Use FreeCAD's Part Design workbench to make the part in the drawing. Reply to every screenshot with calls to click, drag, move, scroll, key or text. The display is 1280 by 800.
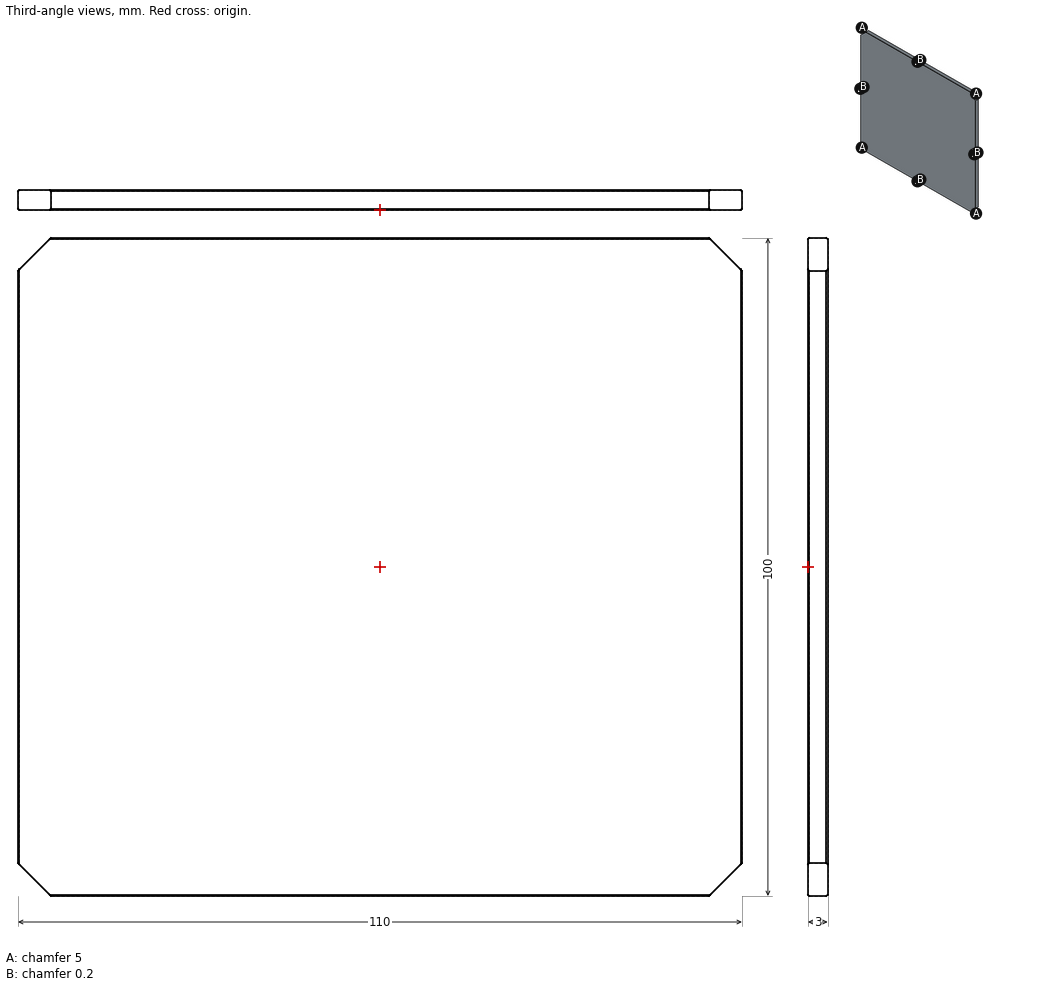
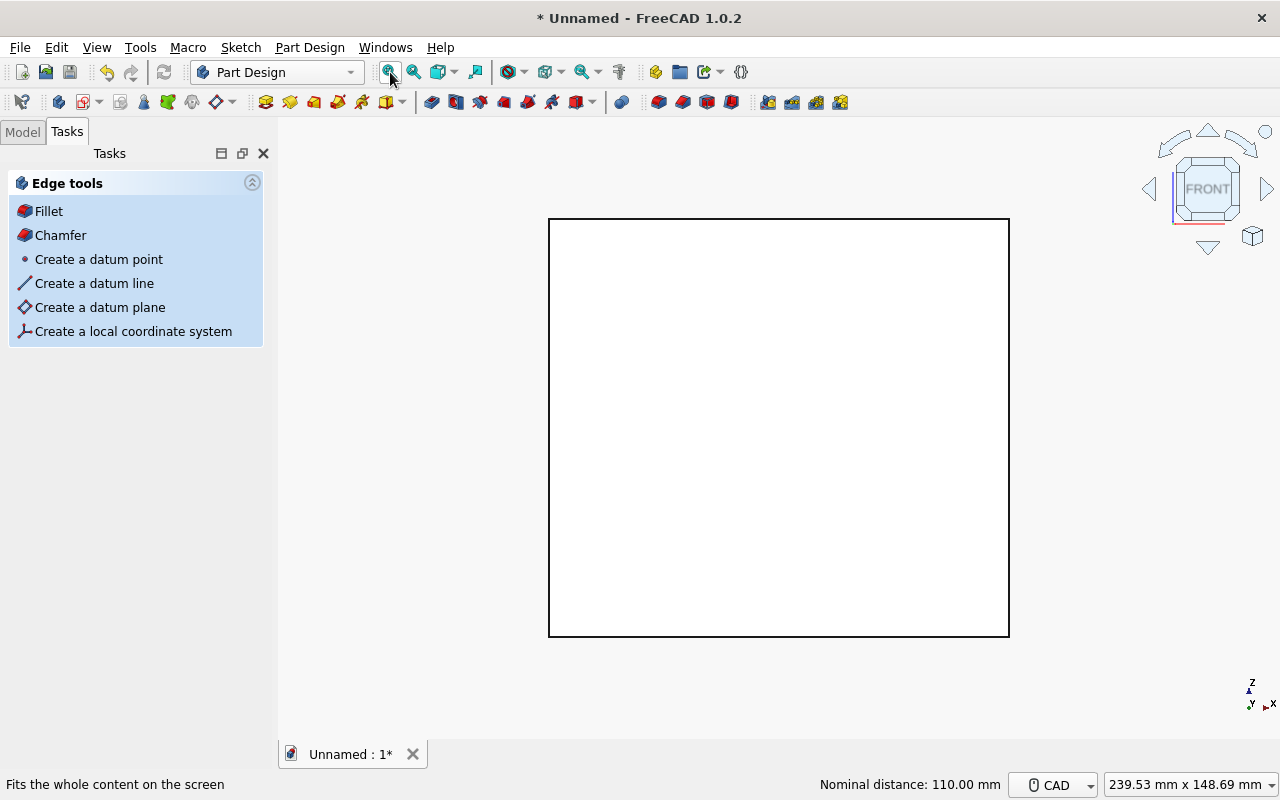
scroll(549, 636, up, 6)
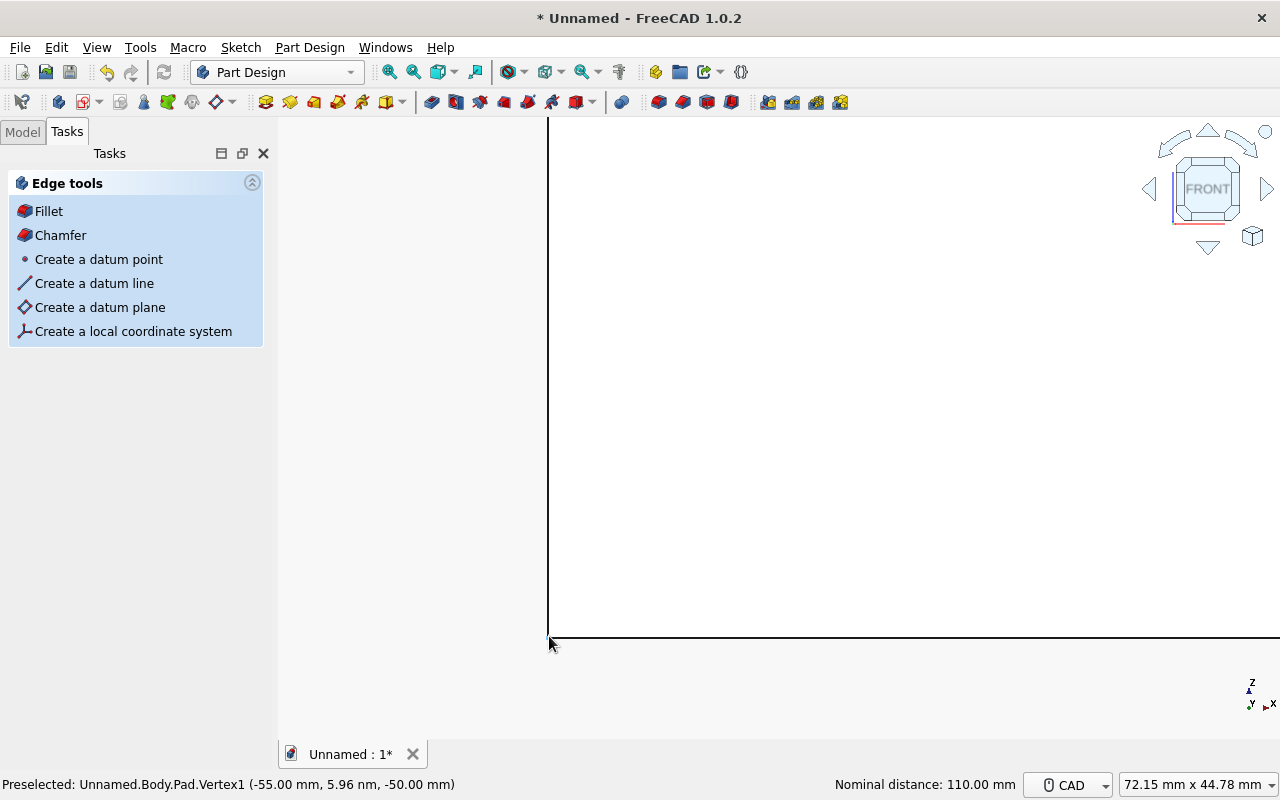
click(390, 72)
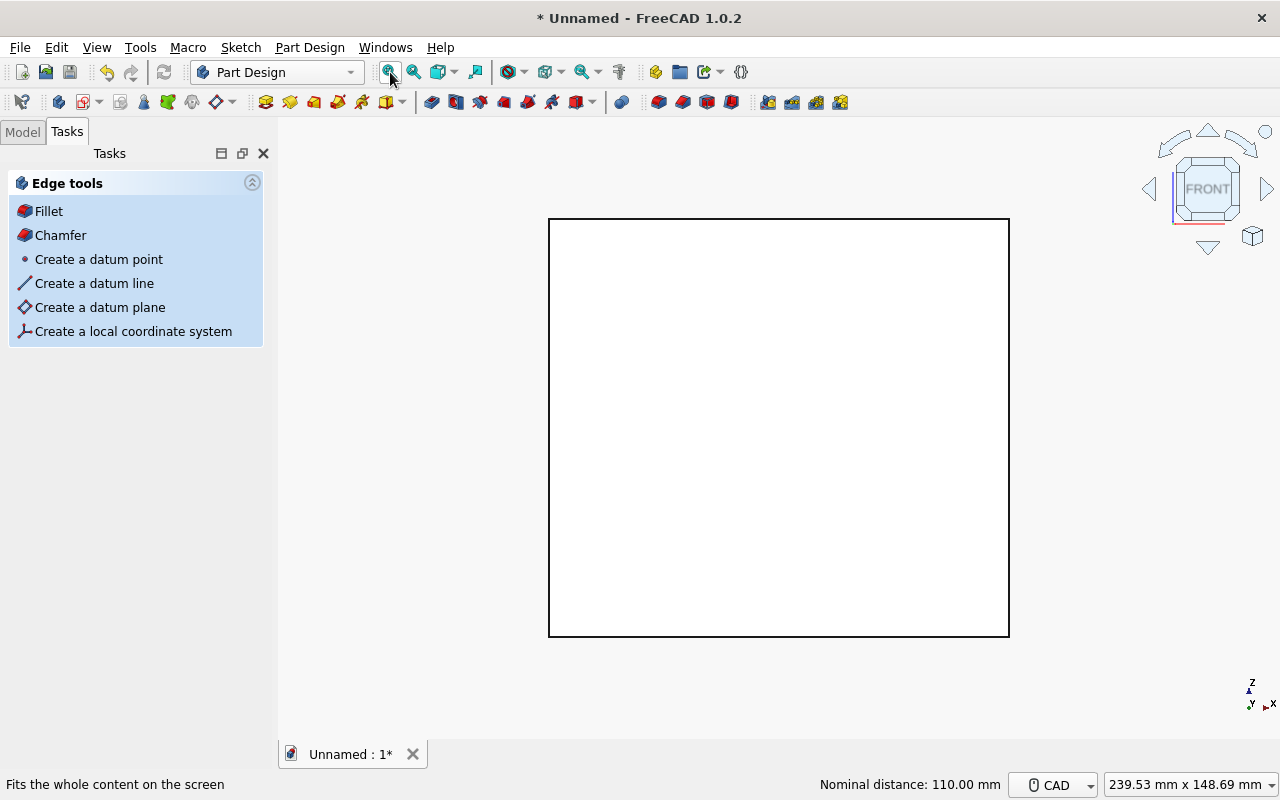
key(3)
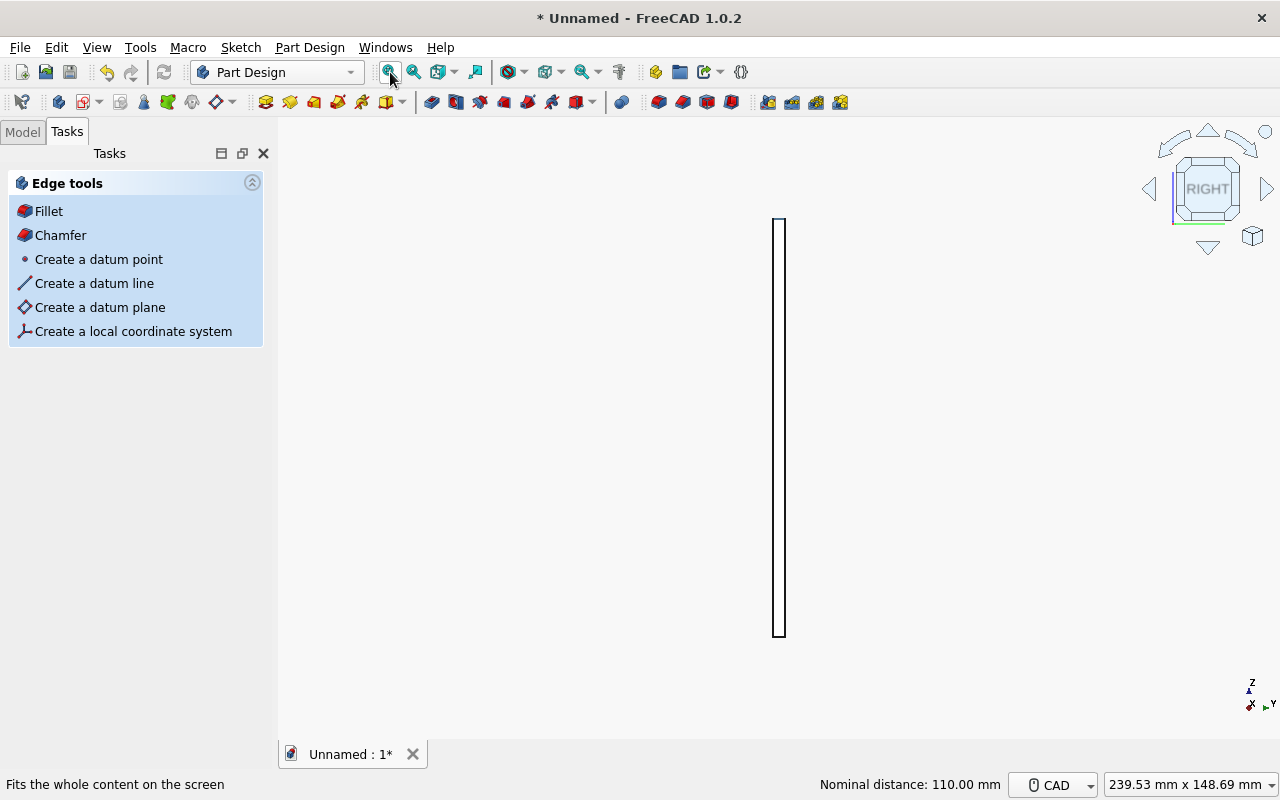
click(779, 636, ctrl)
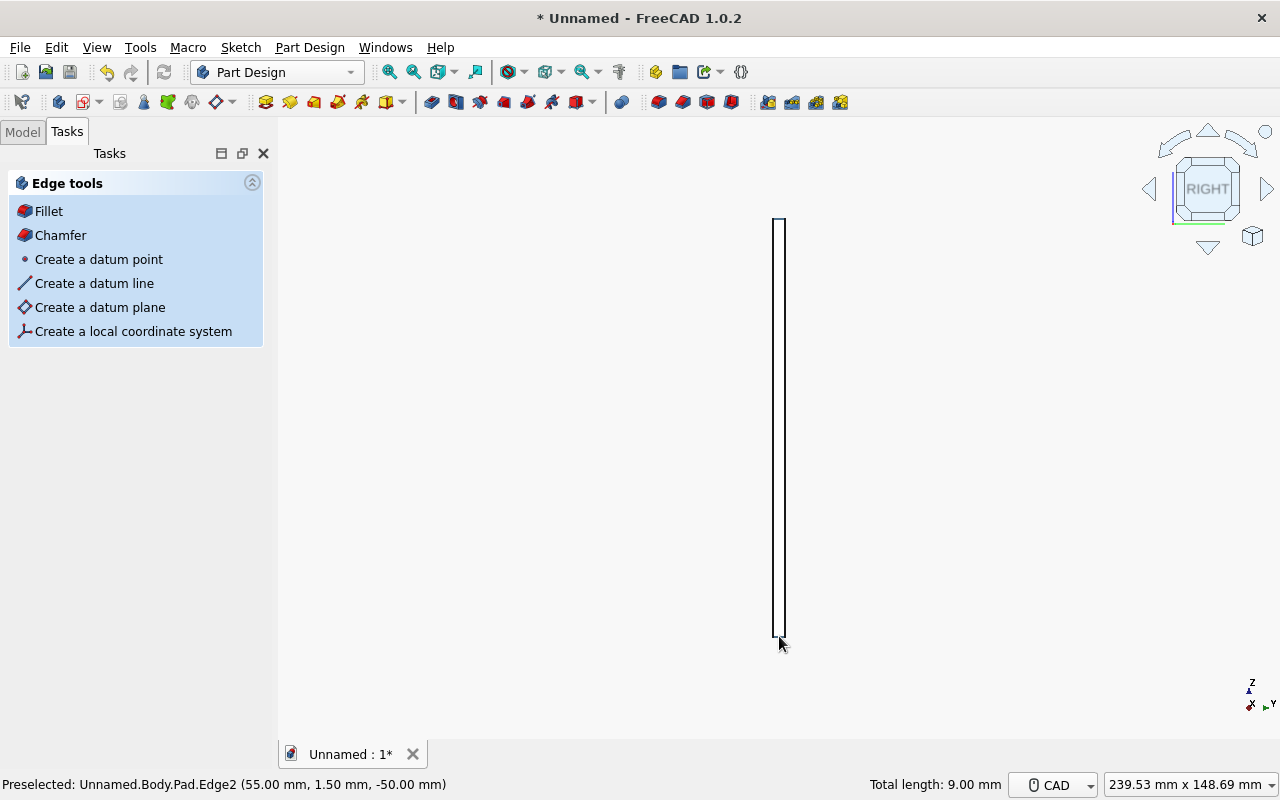
scroll(779, 636, up, 6)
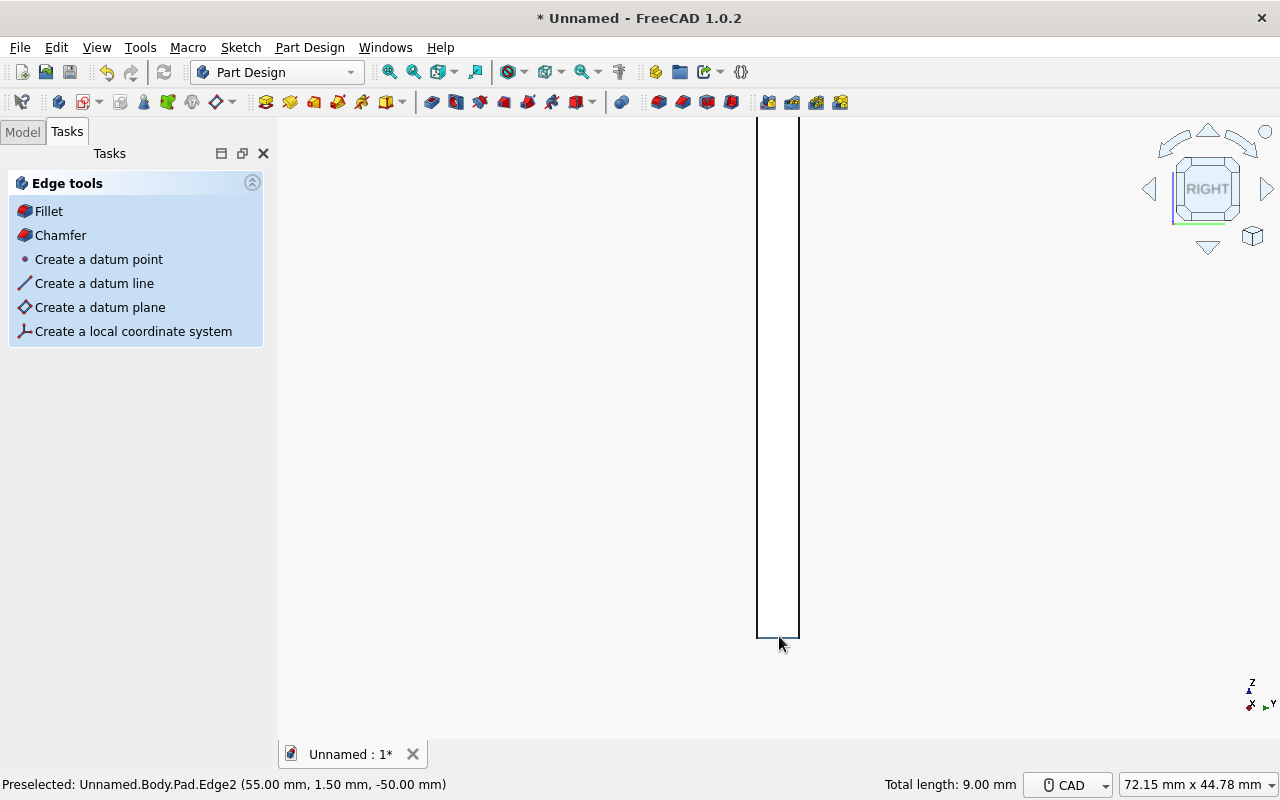
click(390, 72)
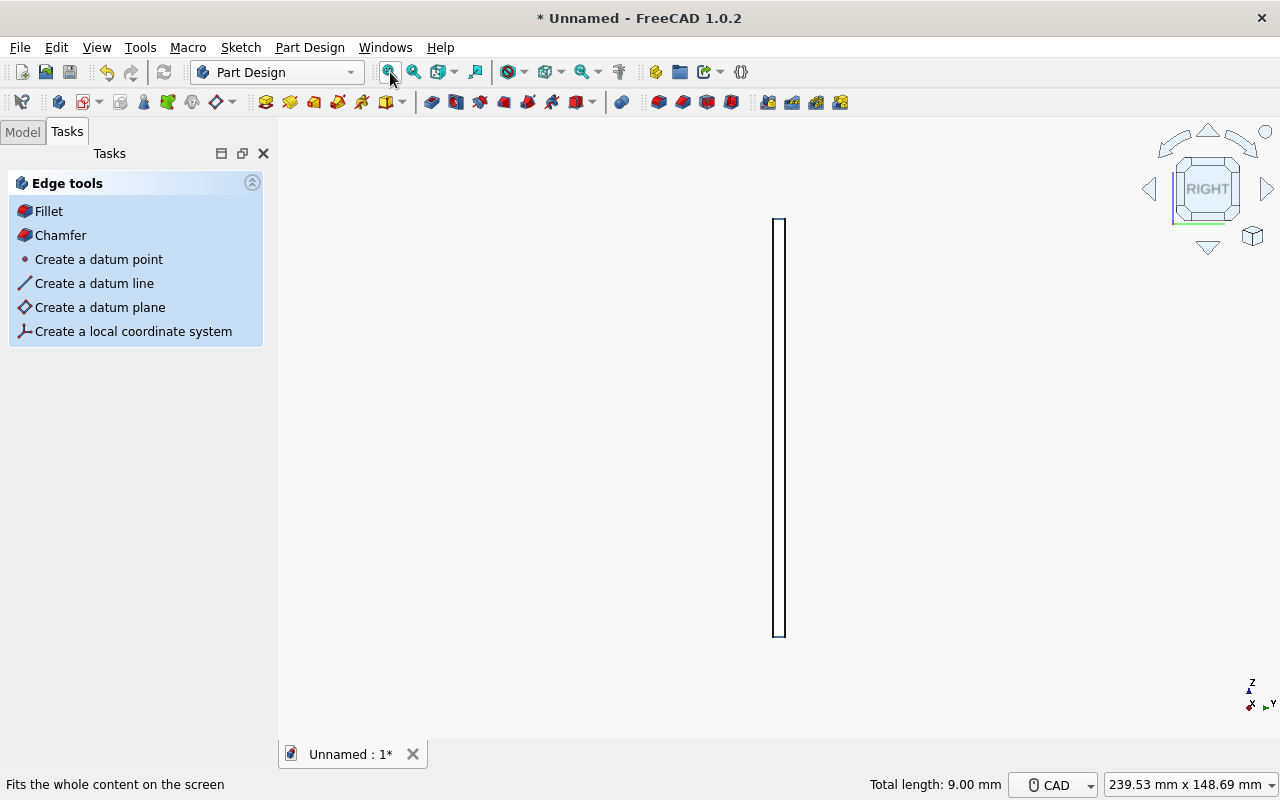
key(5)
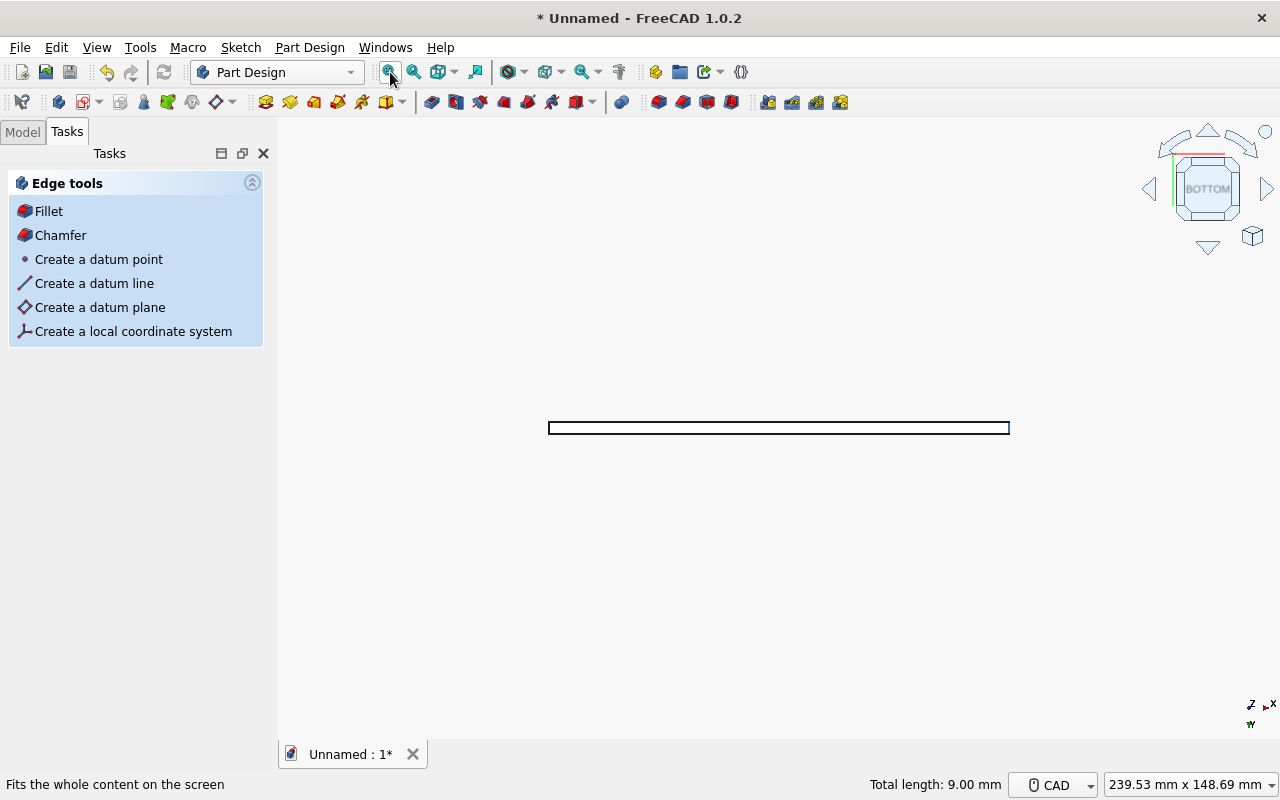
click(549, 427, ctrl)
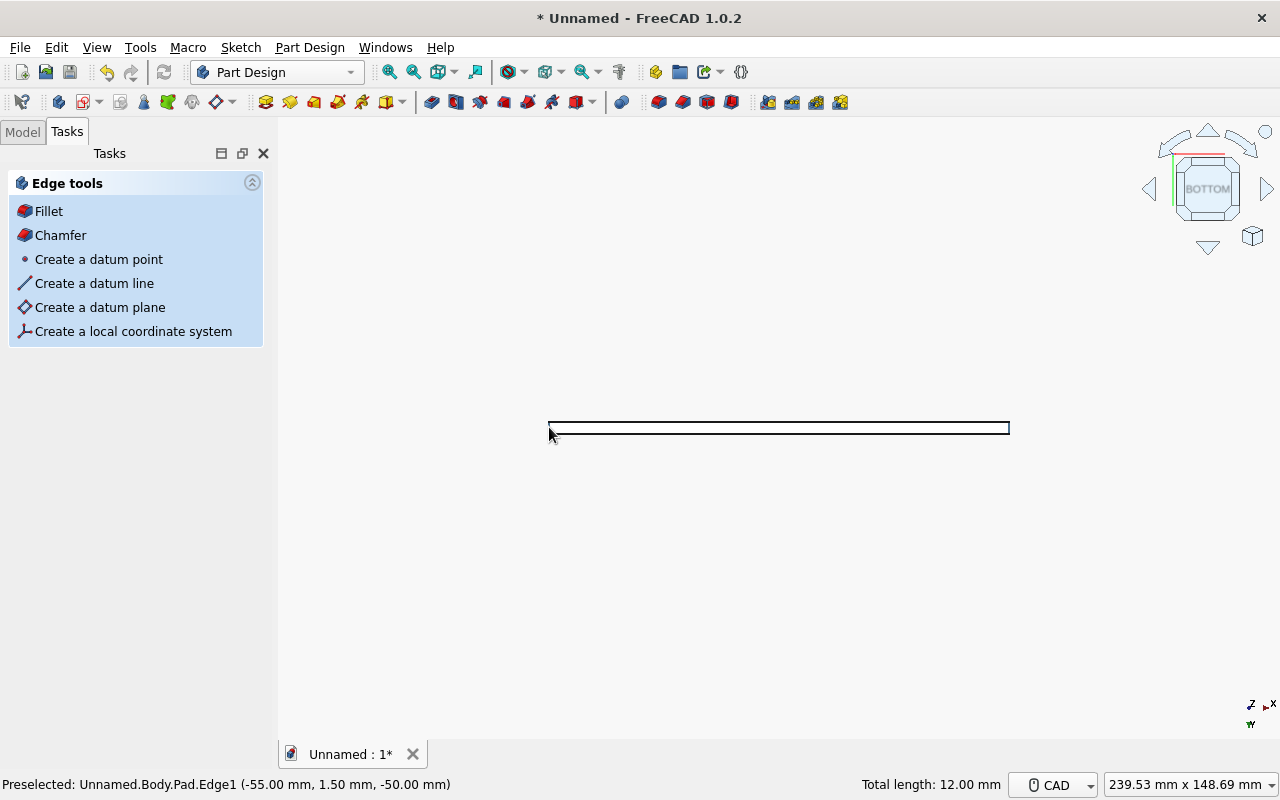
click(684, 102)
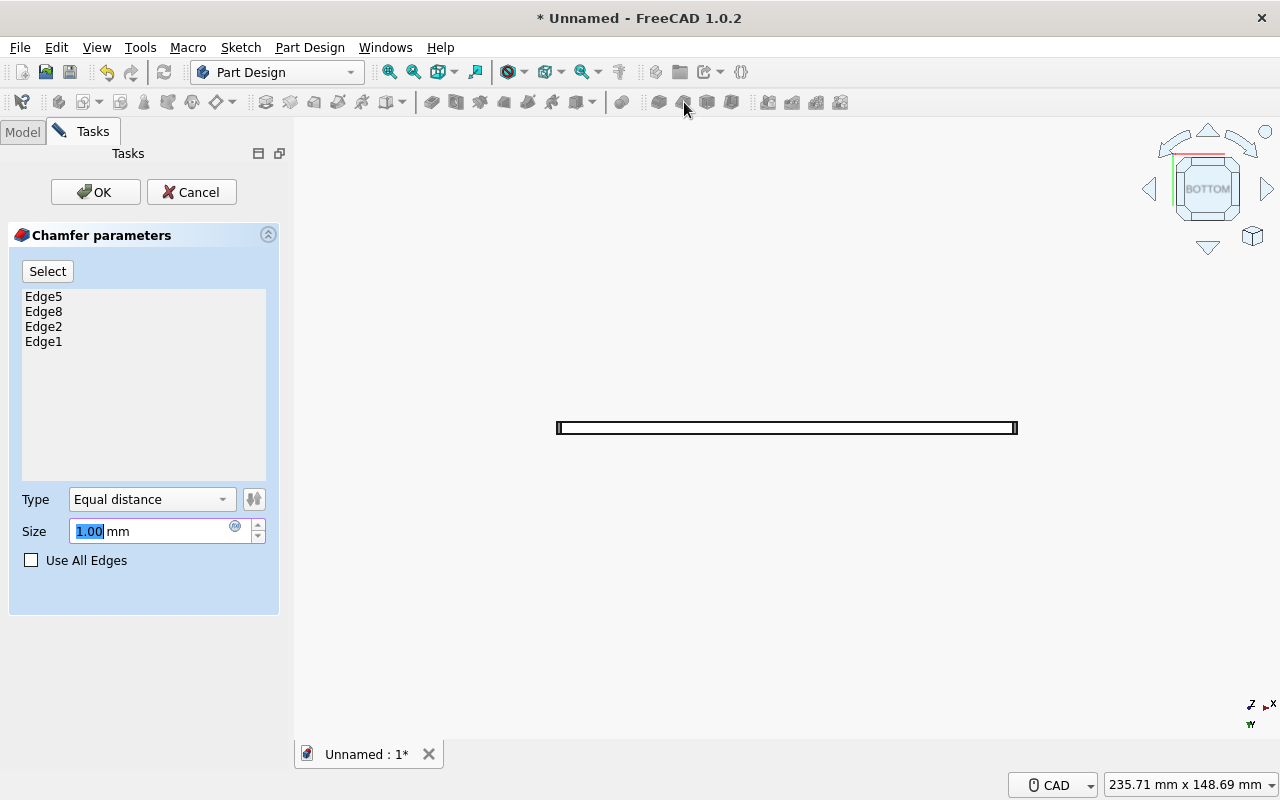
text(5)
key(Tab)